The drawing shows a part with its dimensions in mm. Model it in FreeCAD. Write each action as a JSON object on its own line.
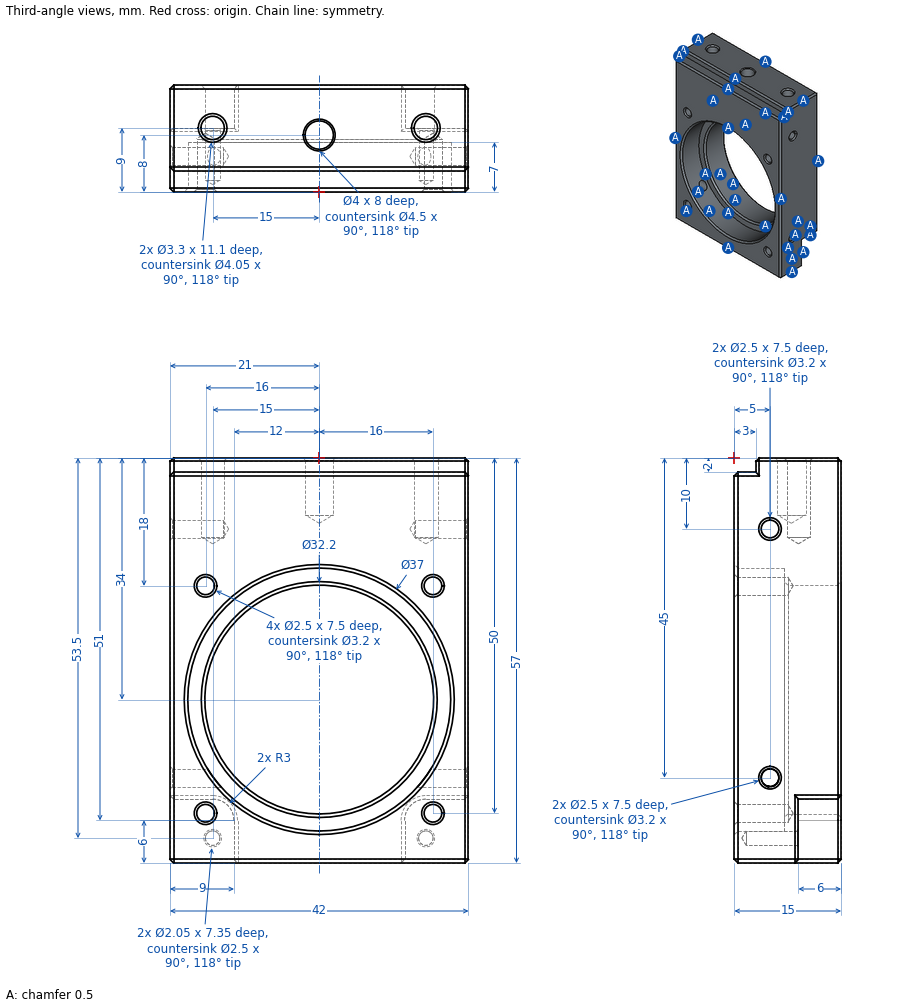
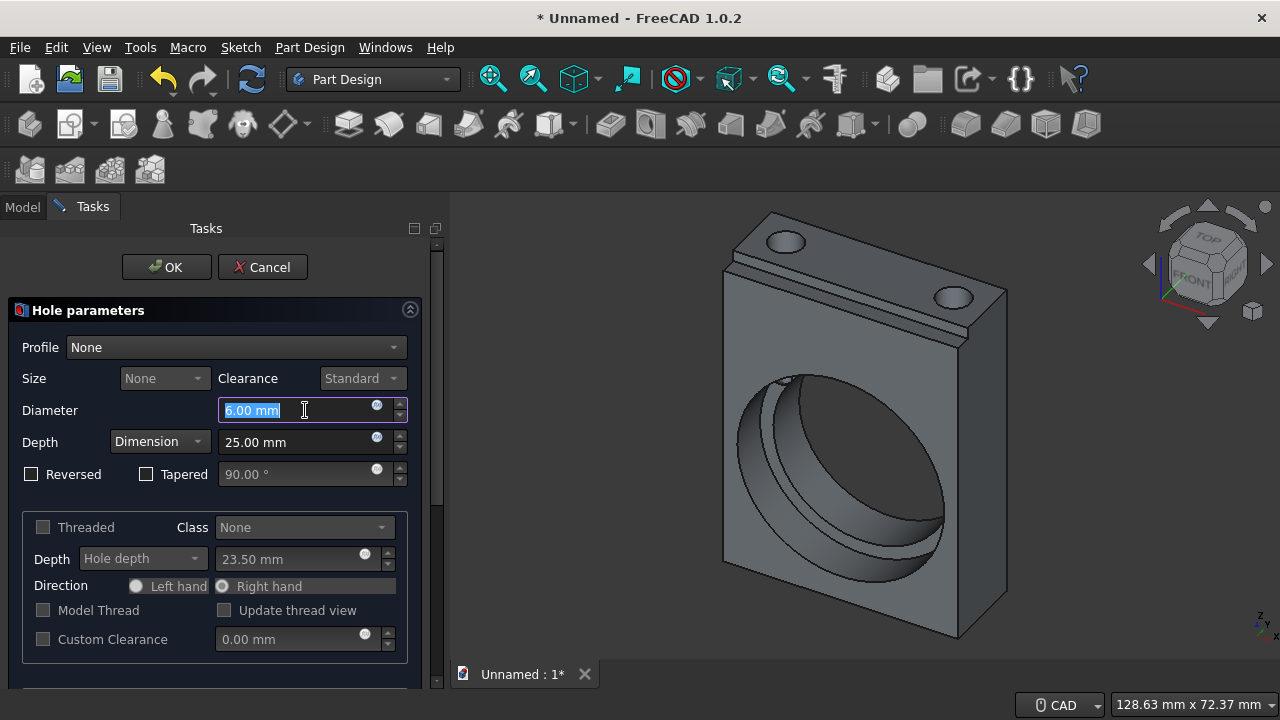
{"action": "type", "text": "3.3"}
{"action": "key", "text": "Tab"}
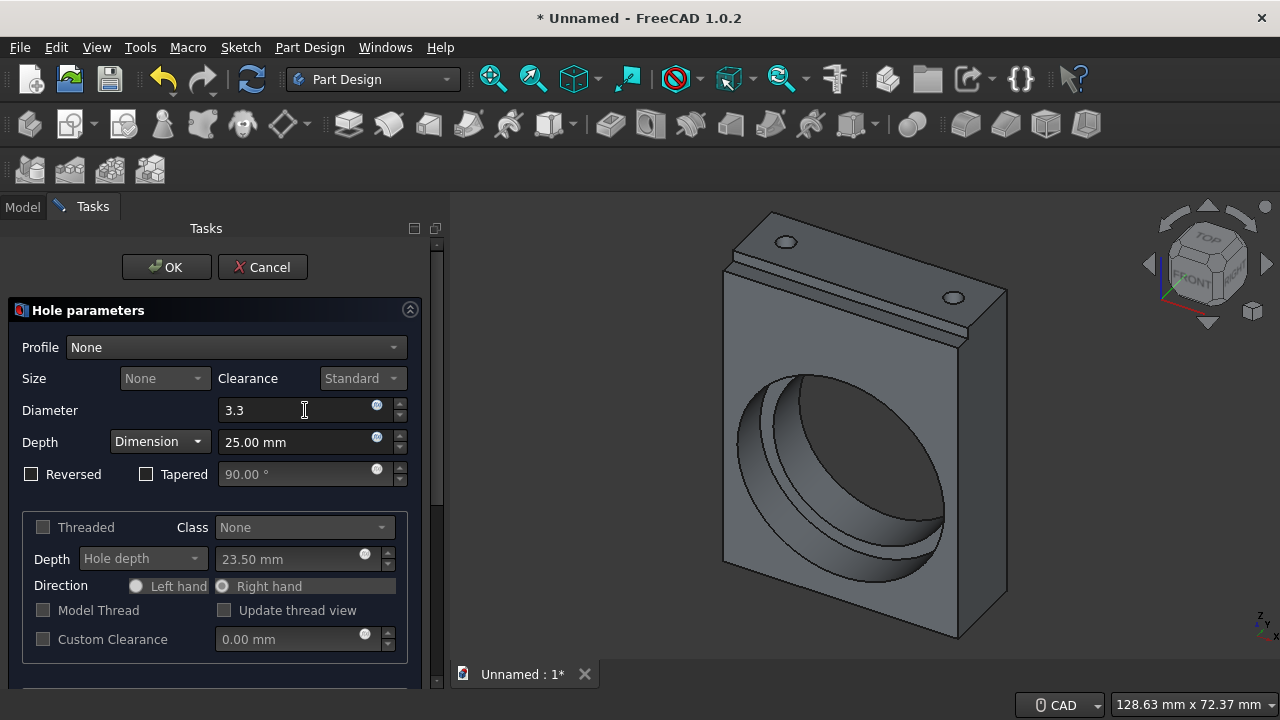
{"action": "triple_click", "coordinate": [305, 442]}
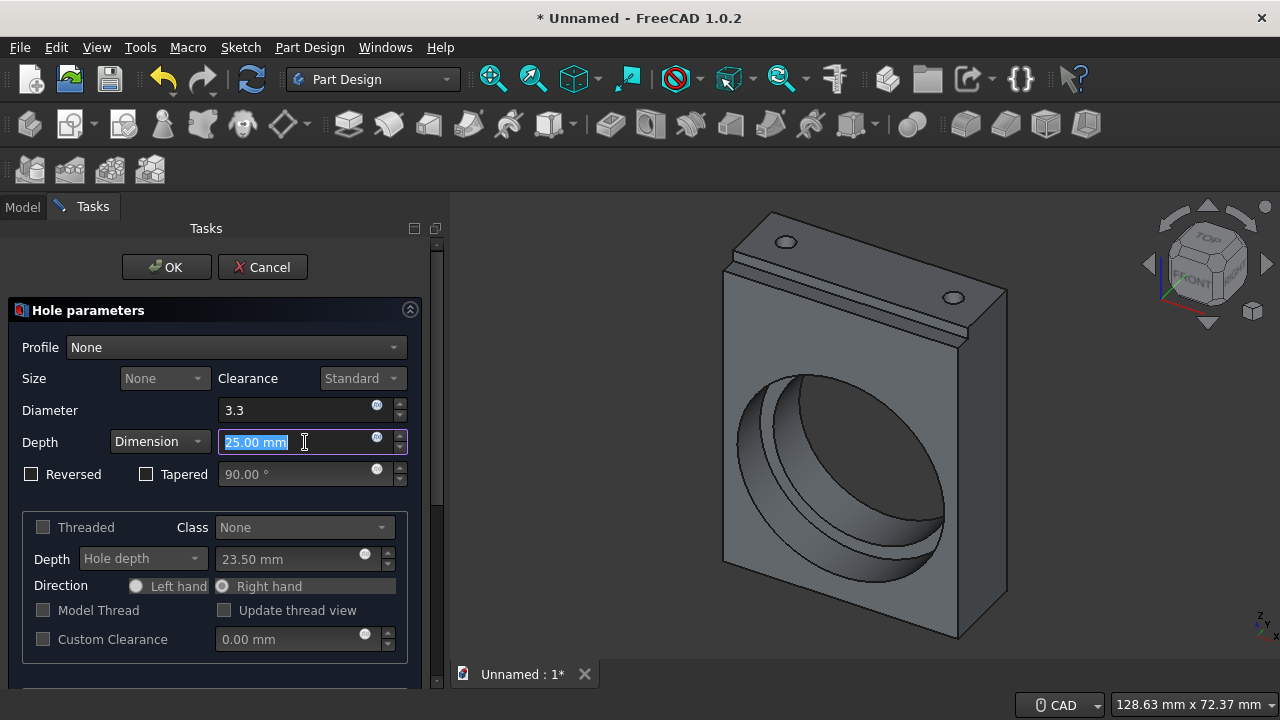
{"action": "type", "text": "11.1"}
{"action": "key", "text": "Tab"}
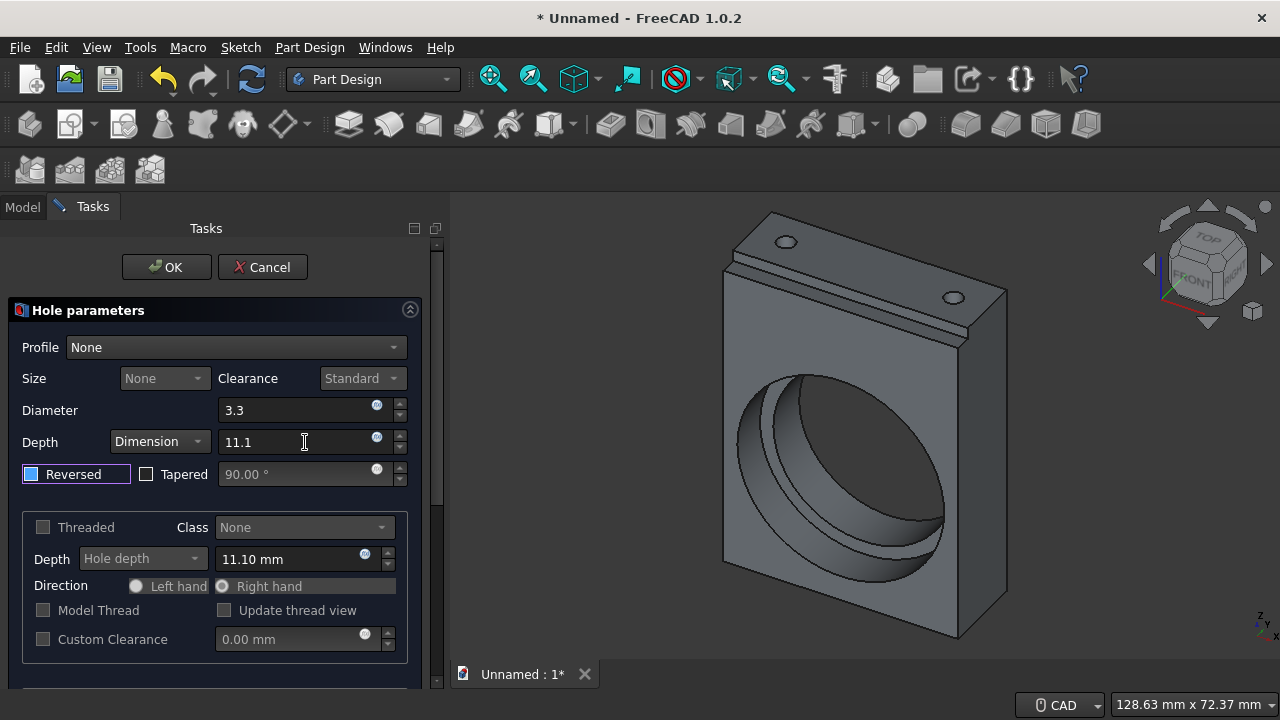
{"action": "scroll", "coordinate": [437, 463], "scroll_direction": "down", "scroll_amount": 2}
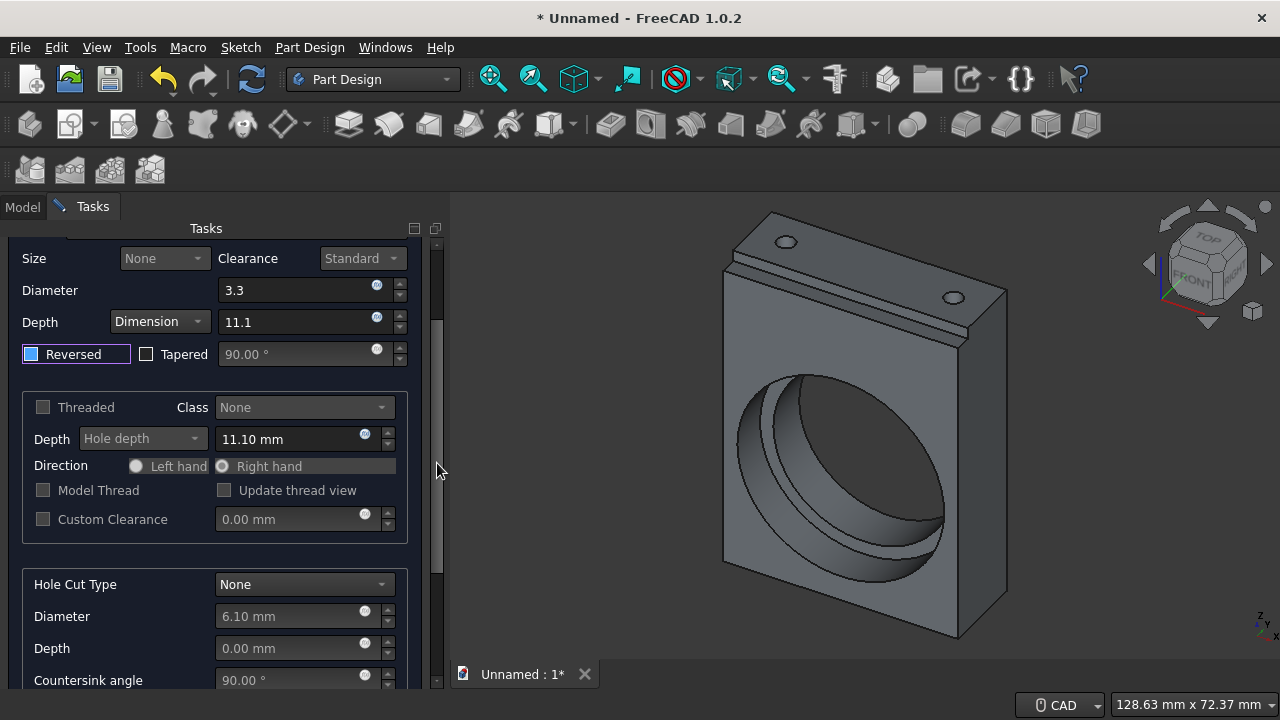
{"action": "left_click", "coordinate": [306, 584]}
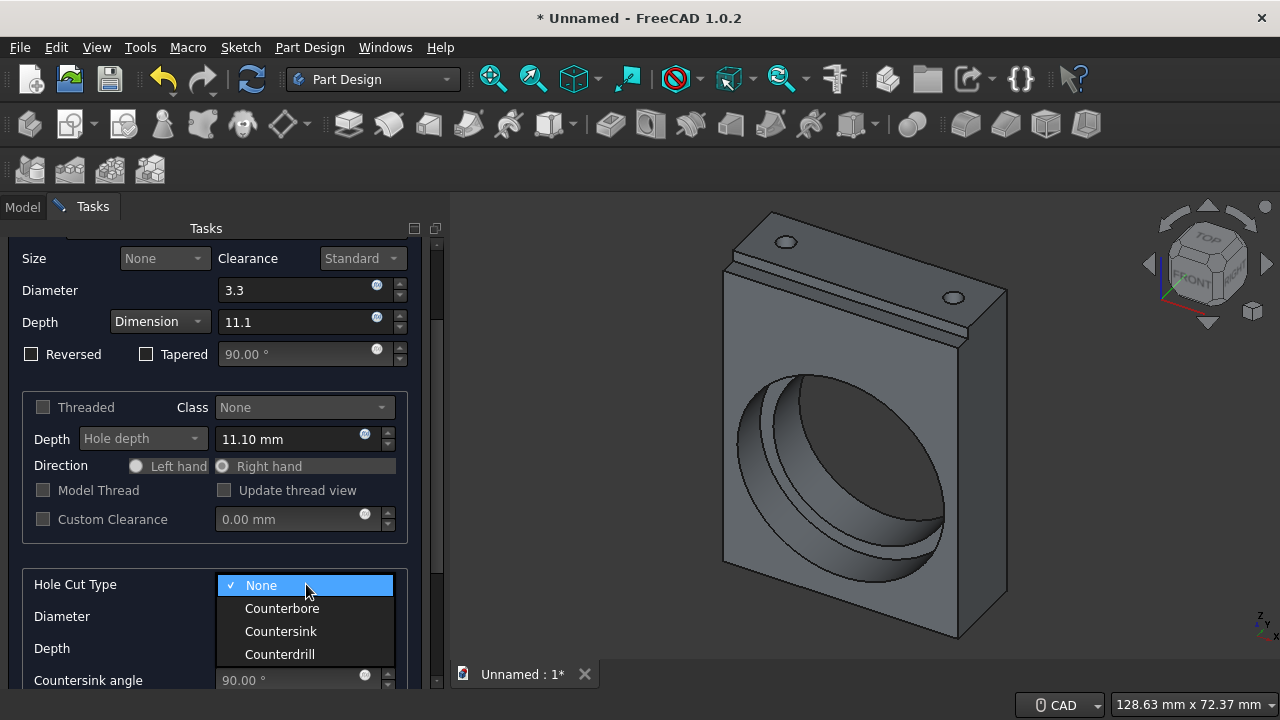
{"action": "left_click", "coordinate": [304, 632]}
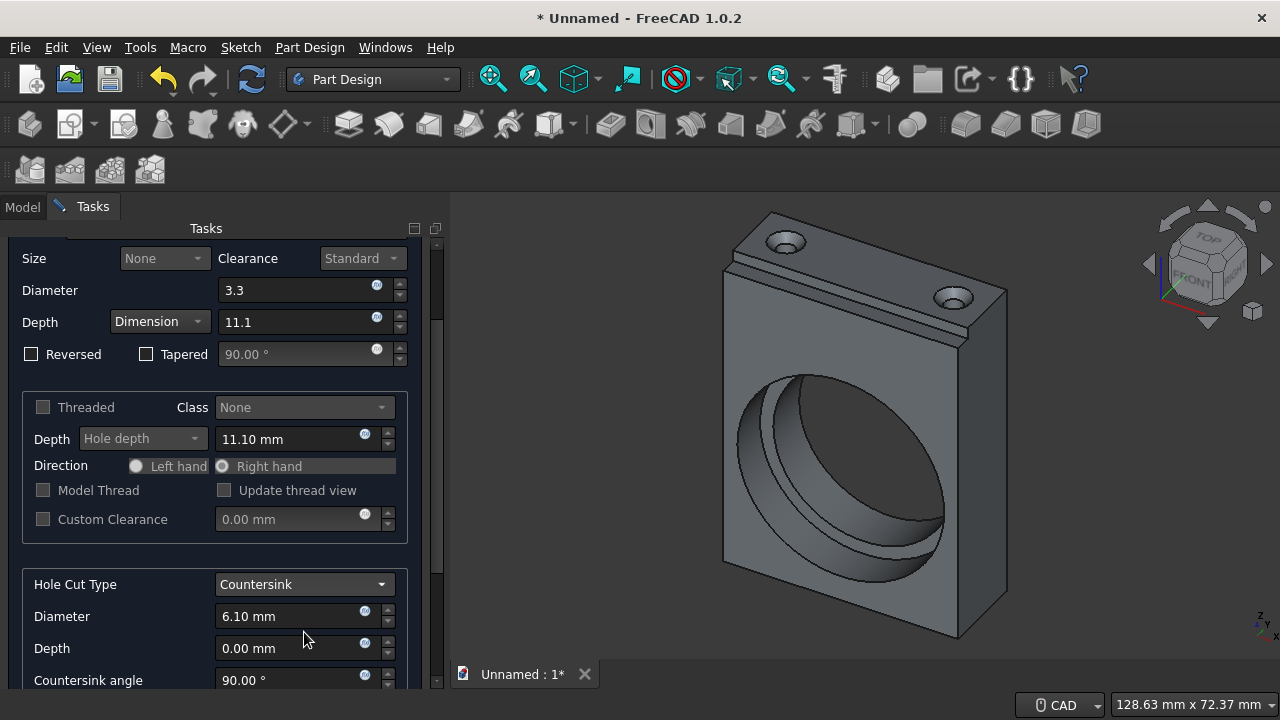
{"action": "triple_click", "coordinate": [298, 616]}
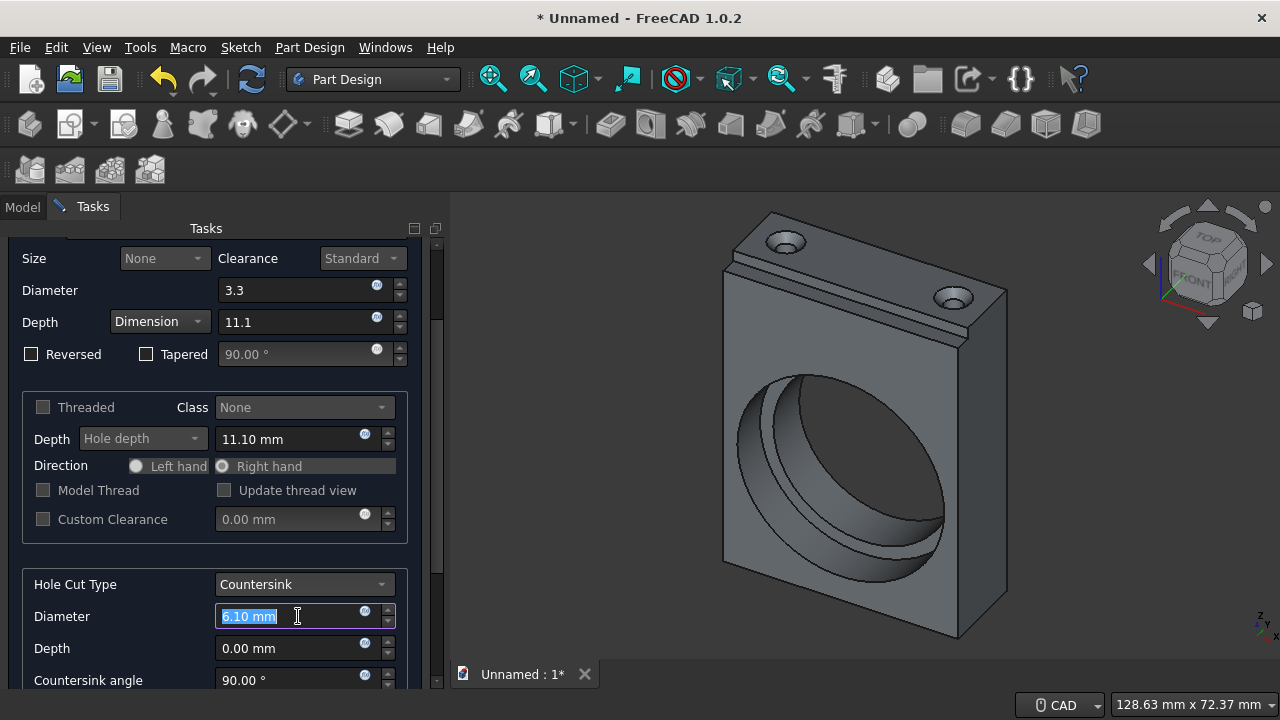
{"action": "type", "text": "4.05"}
{"action": "key", "text": "Tab"}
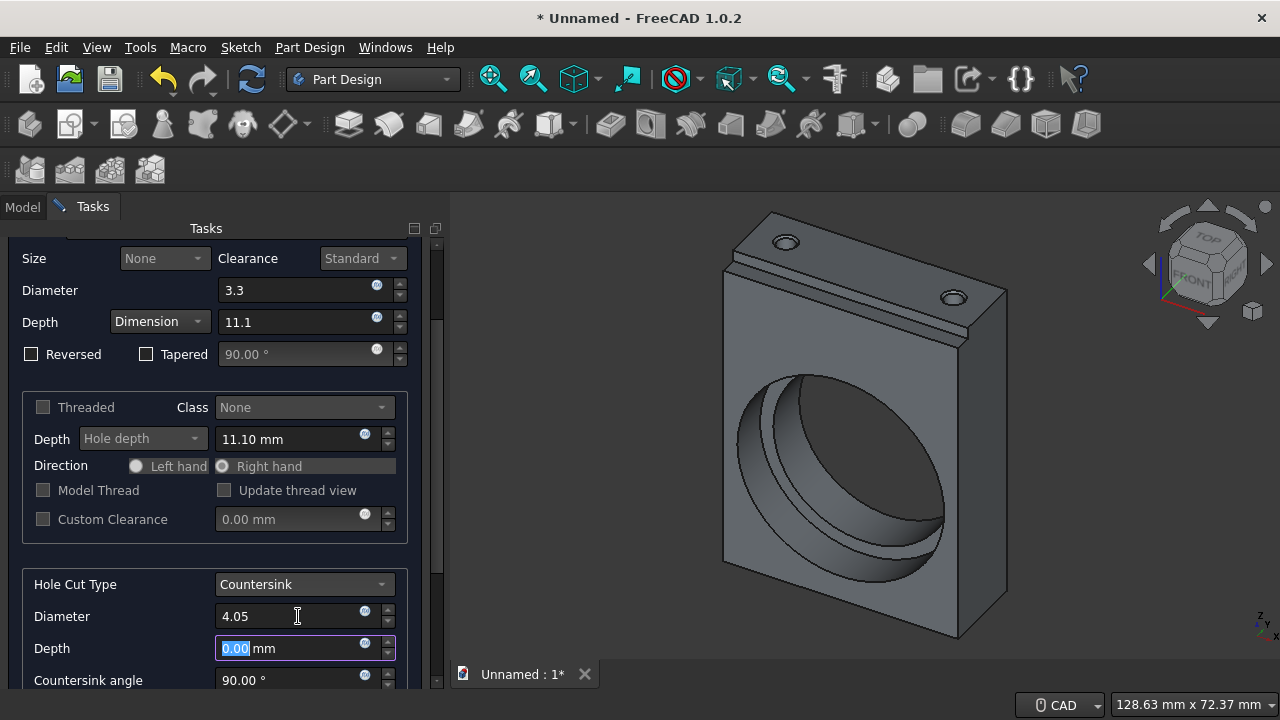
{"action": "scroll", "coordinate": [437, 463], "scroll_direction": "up", "scroll_amount": 3}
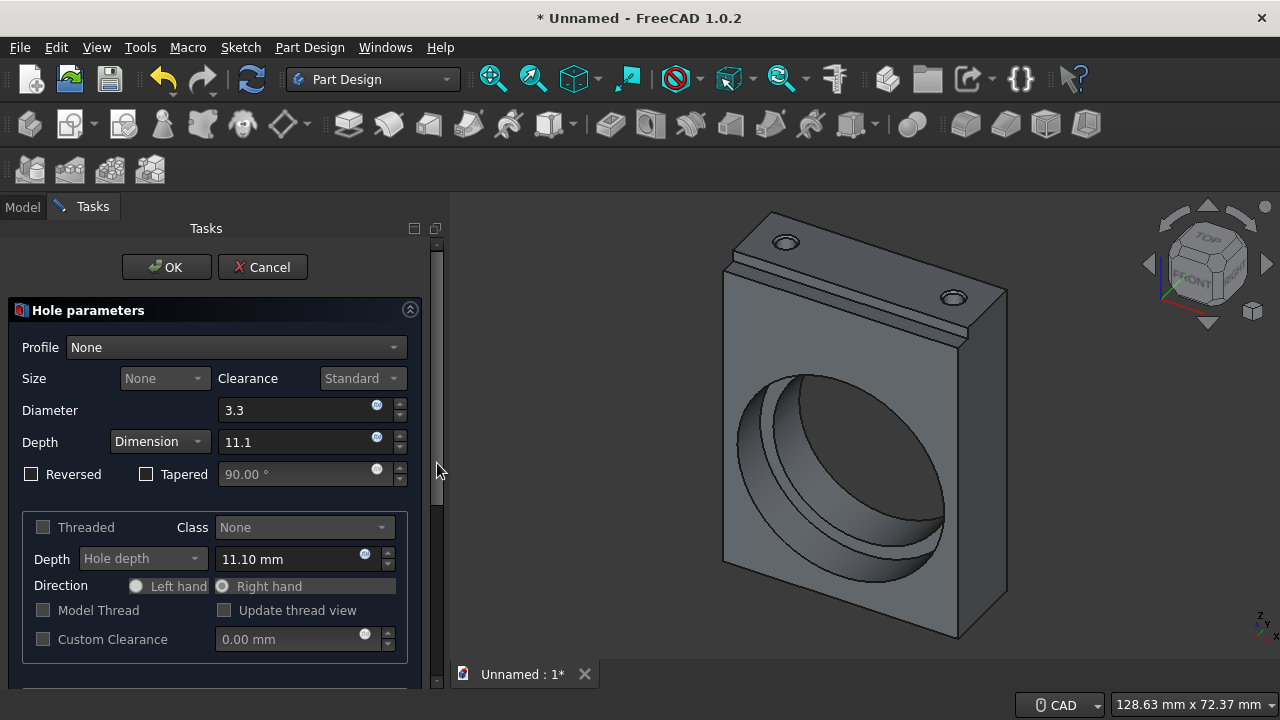
{"action": "left_click", "coordinate": [167, 267]}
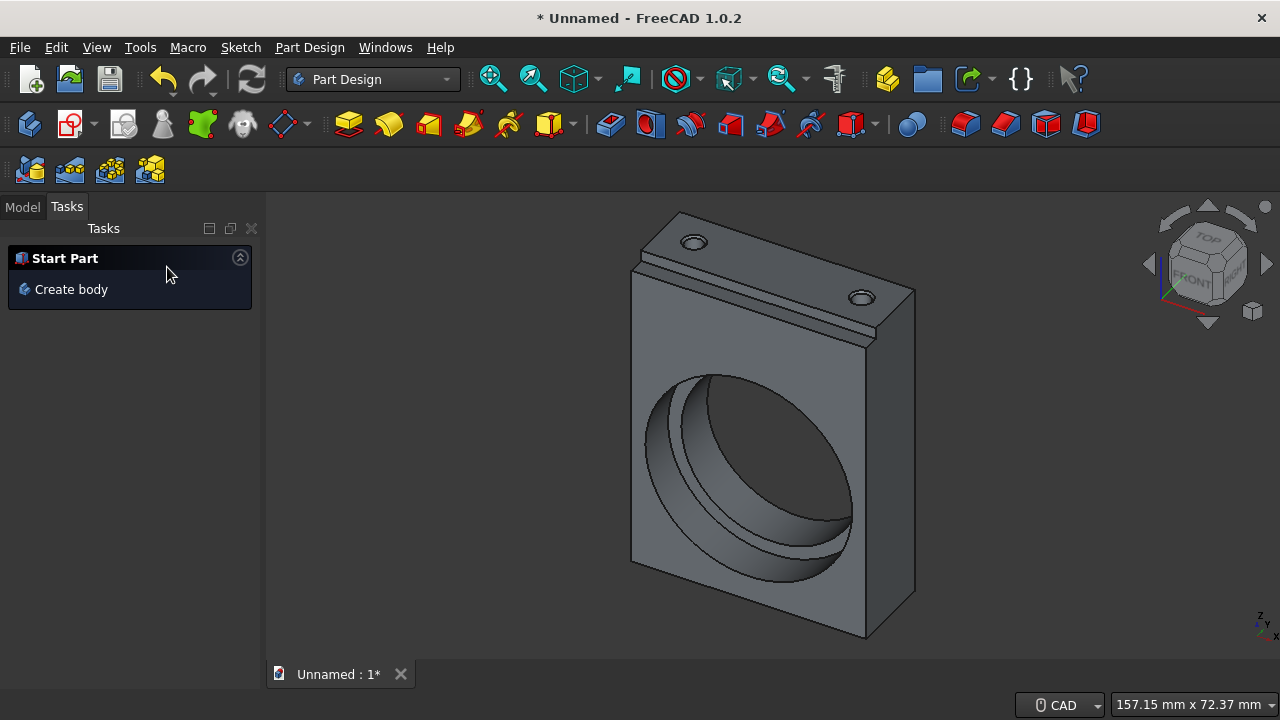
{"action": "left_click", "coordinate": [70, 124]}